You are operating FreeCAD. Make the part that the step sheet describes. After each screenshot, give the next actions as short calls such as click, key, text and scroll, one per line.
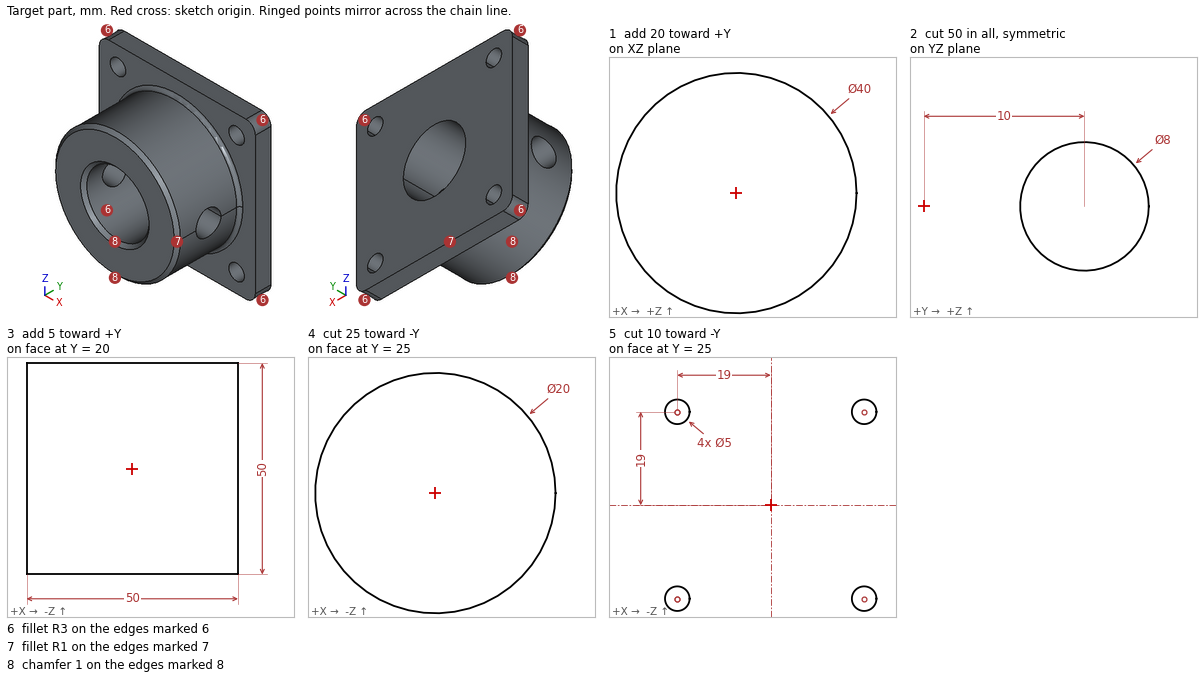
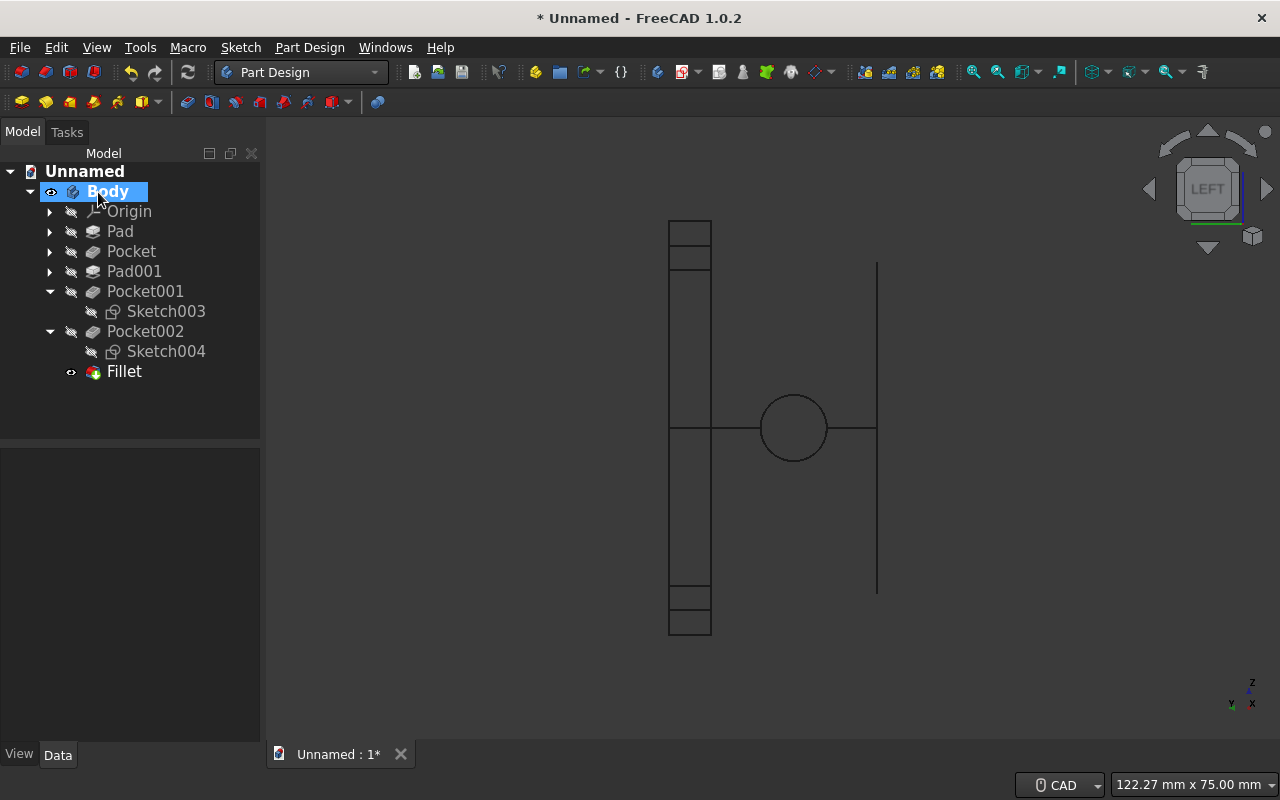
key(0)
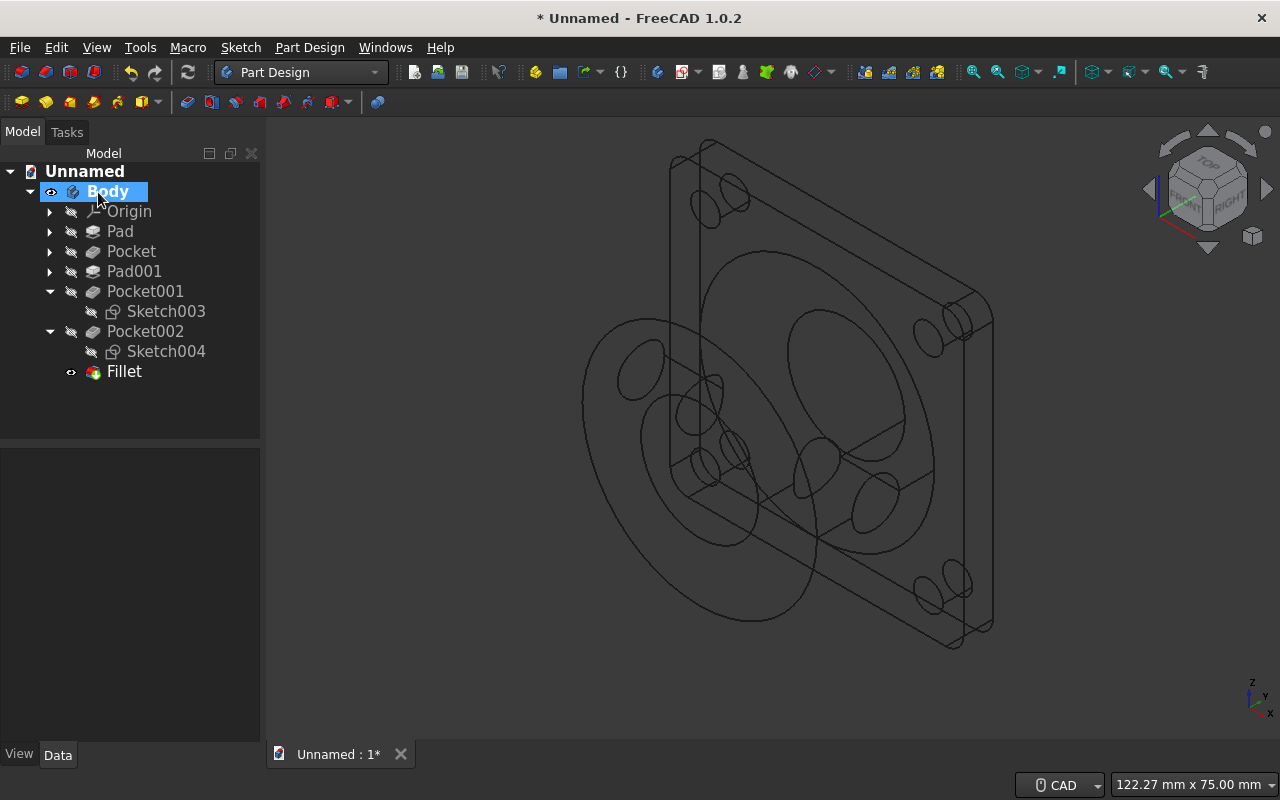
click(722, 267)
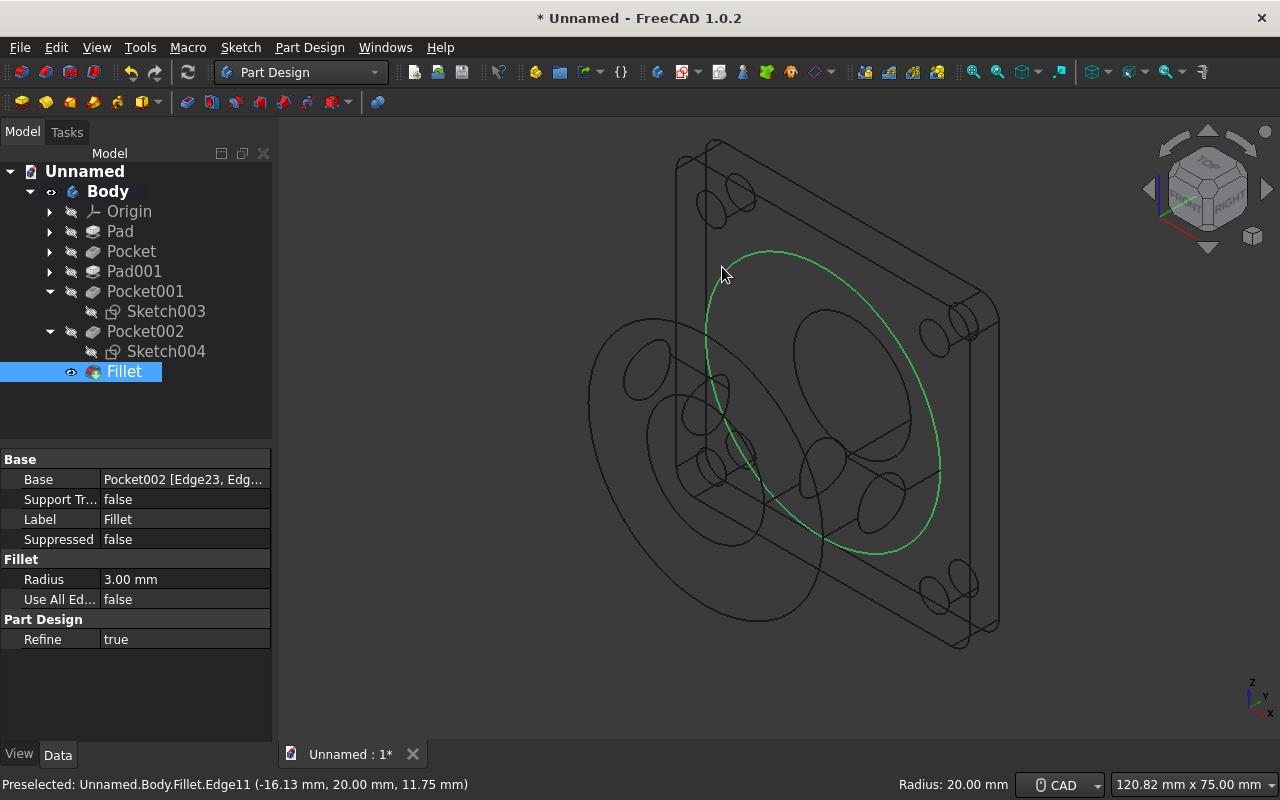
key(v)
key(1)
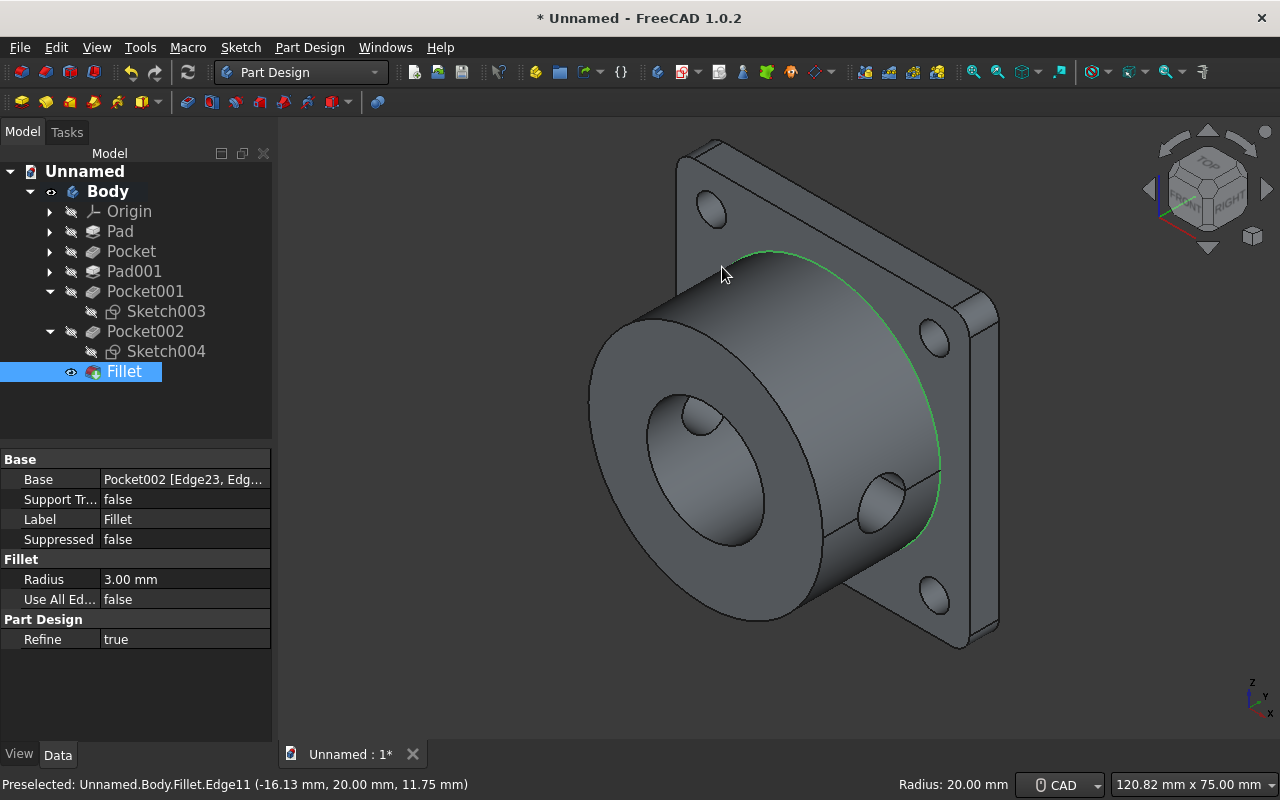
click(22, 72)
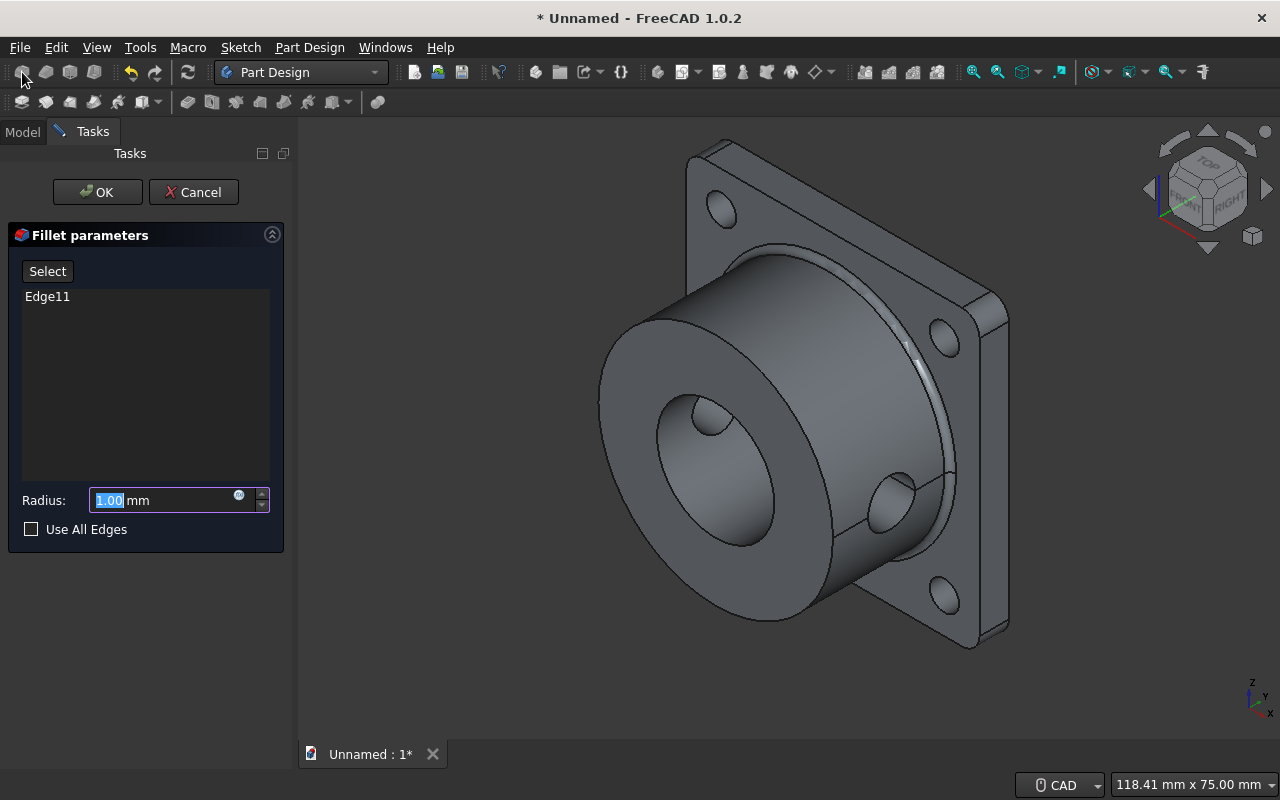
text(1)
key(Tab)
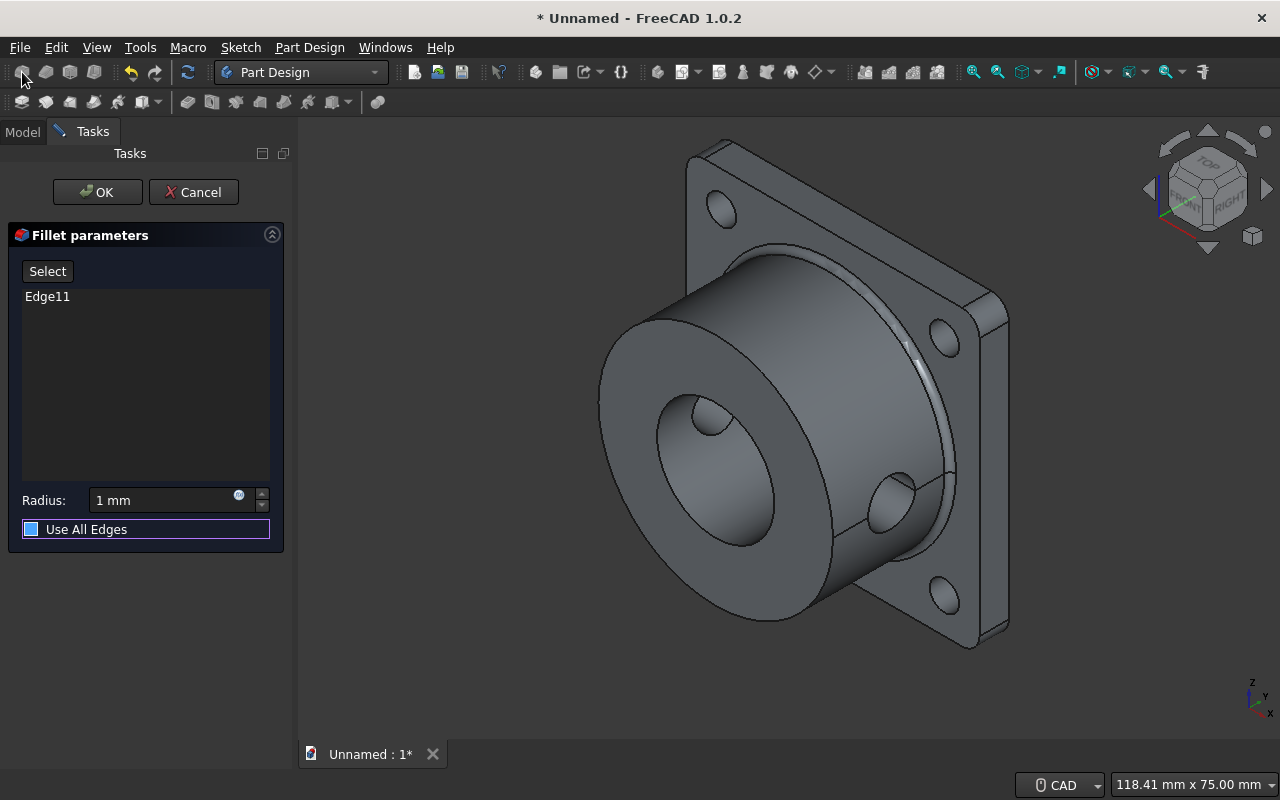
click(98, 192)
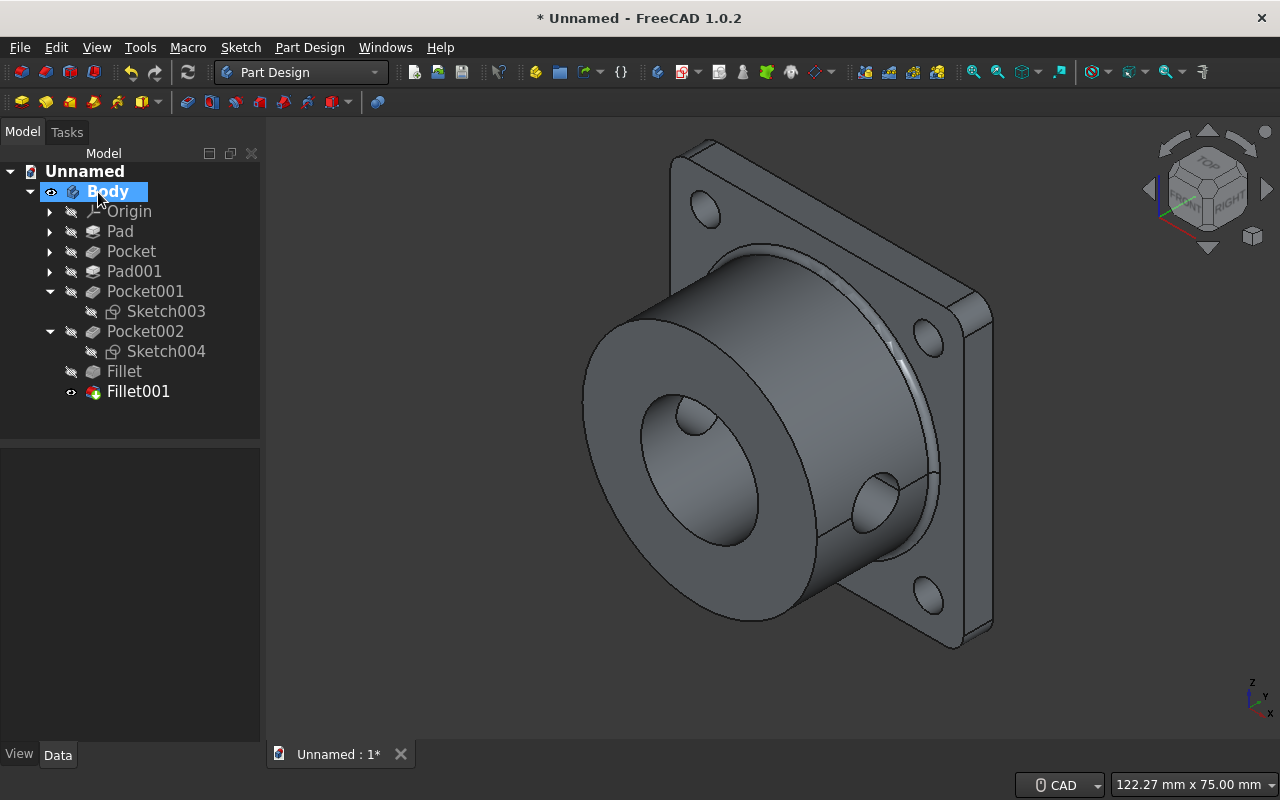
click(605, 335)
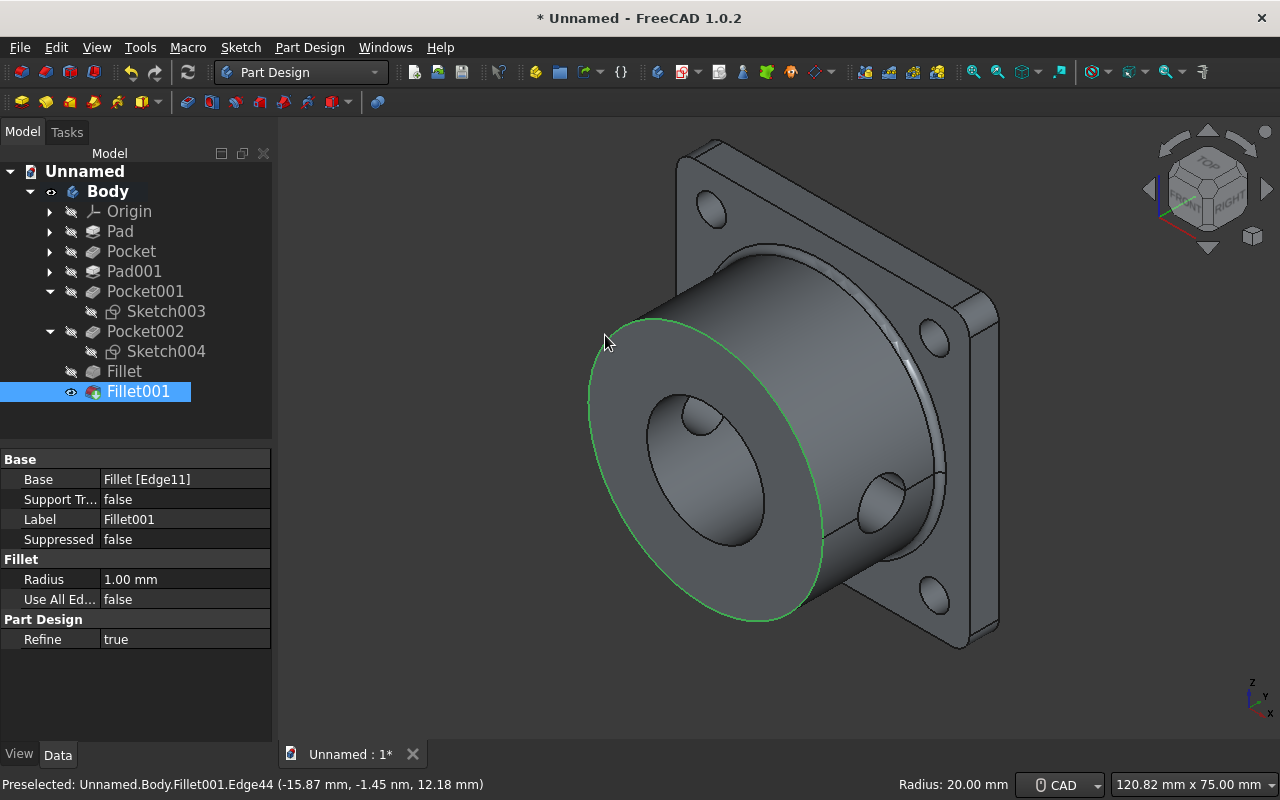
click(647, 435, ctrl)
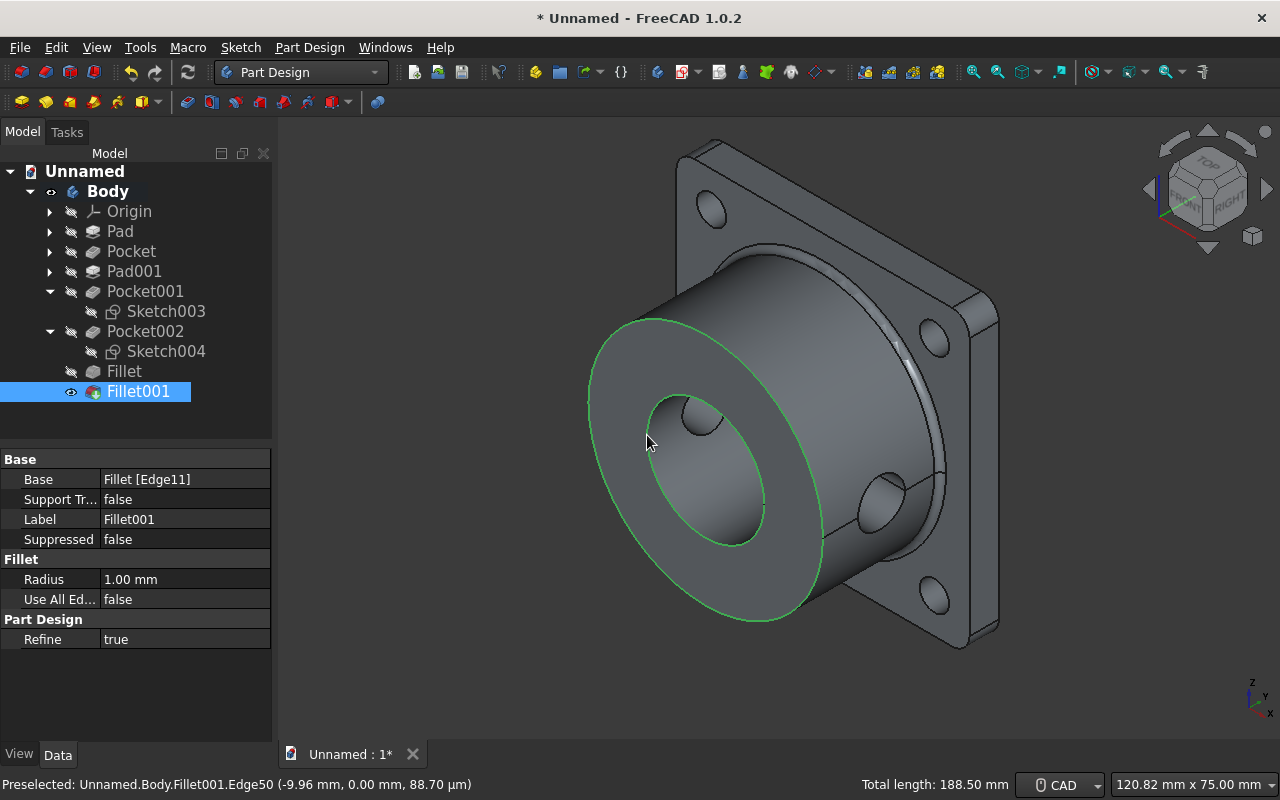
click(46, 72)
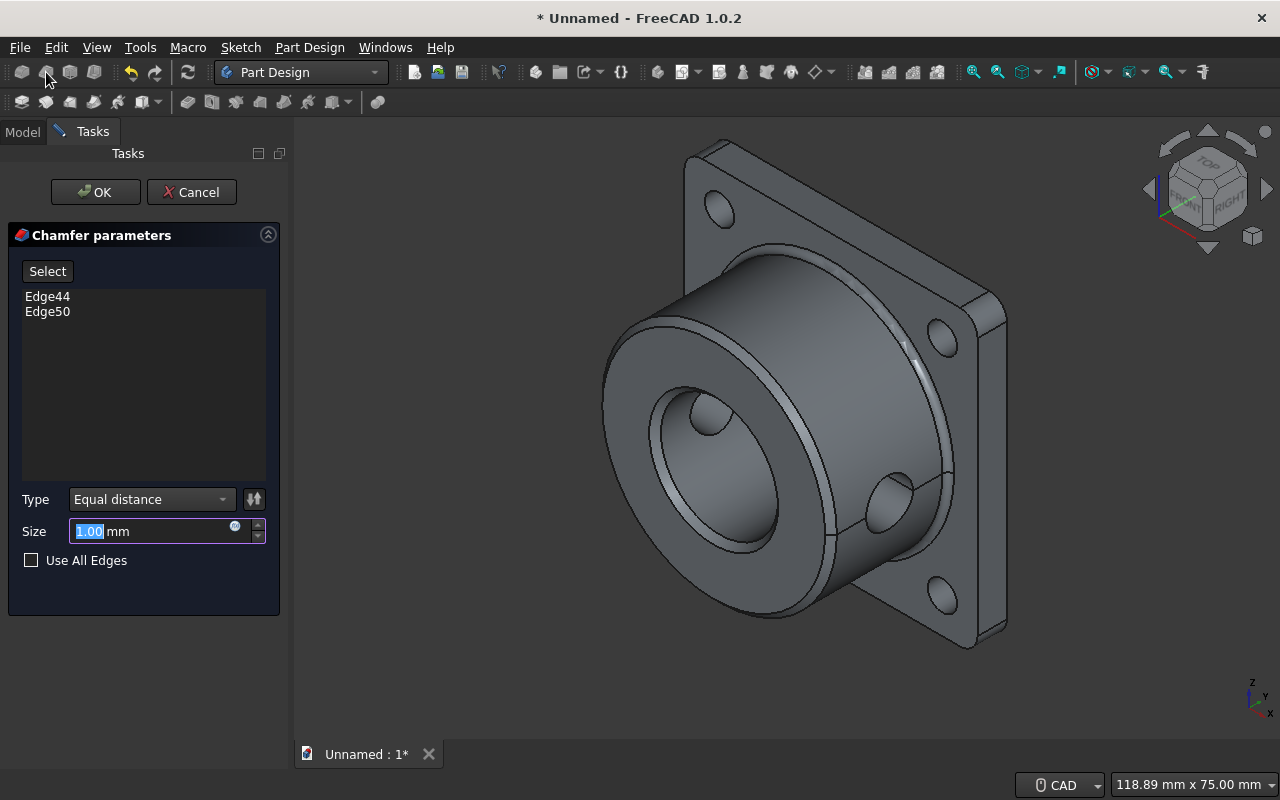
text(1)
key(Tab)